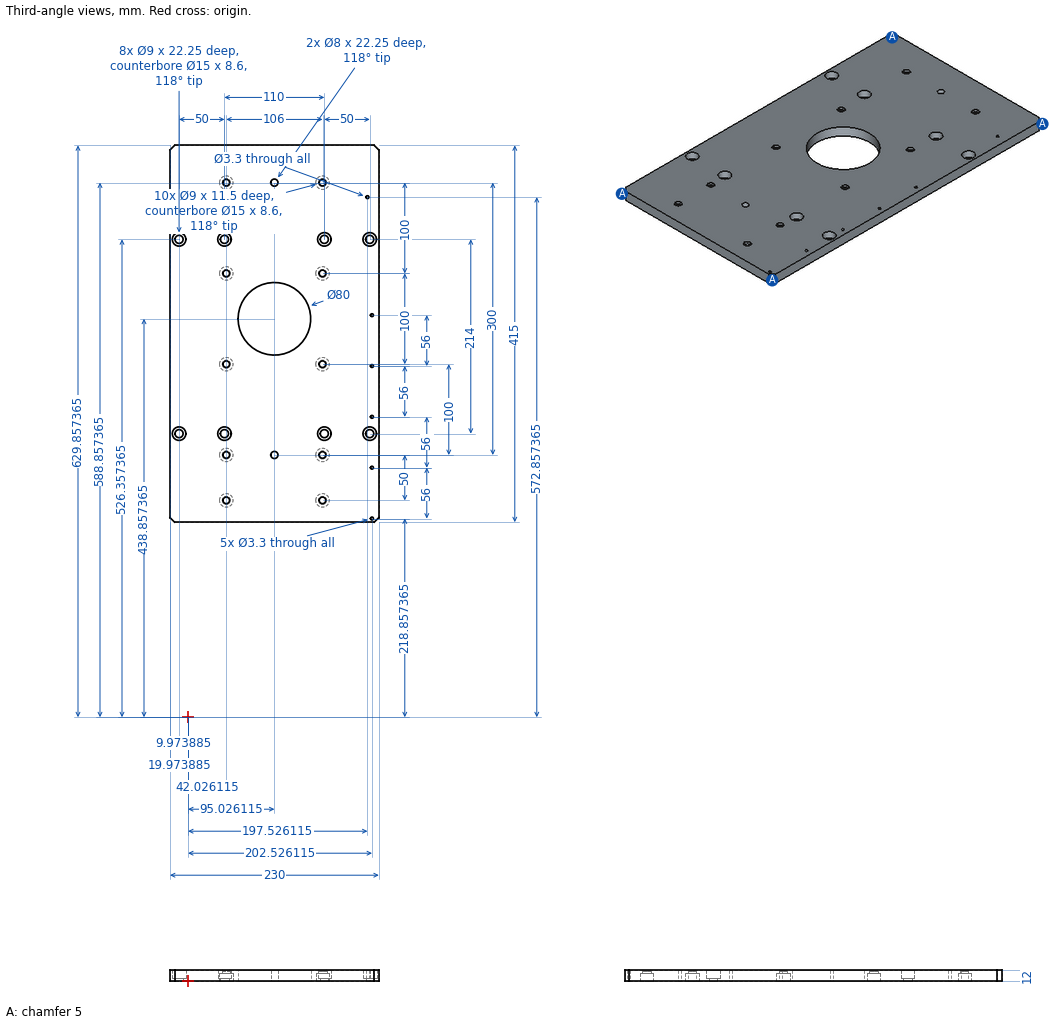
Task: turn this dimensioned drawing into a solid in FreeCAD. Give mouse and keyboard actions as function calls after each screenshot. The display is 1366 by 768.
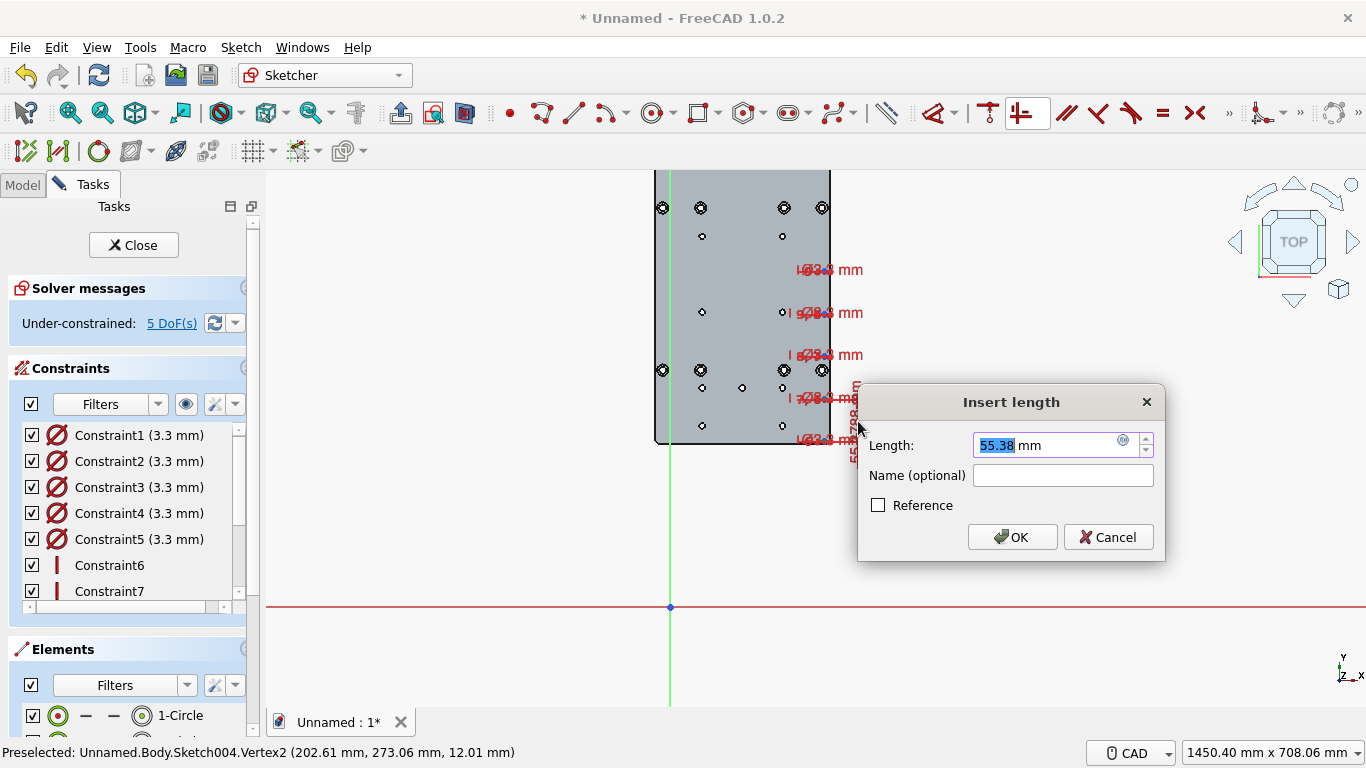
text(56)
key(Return)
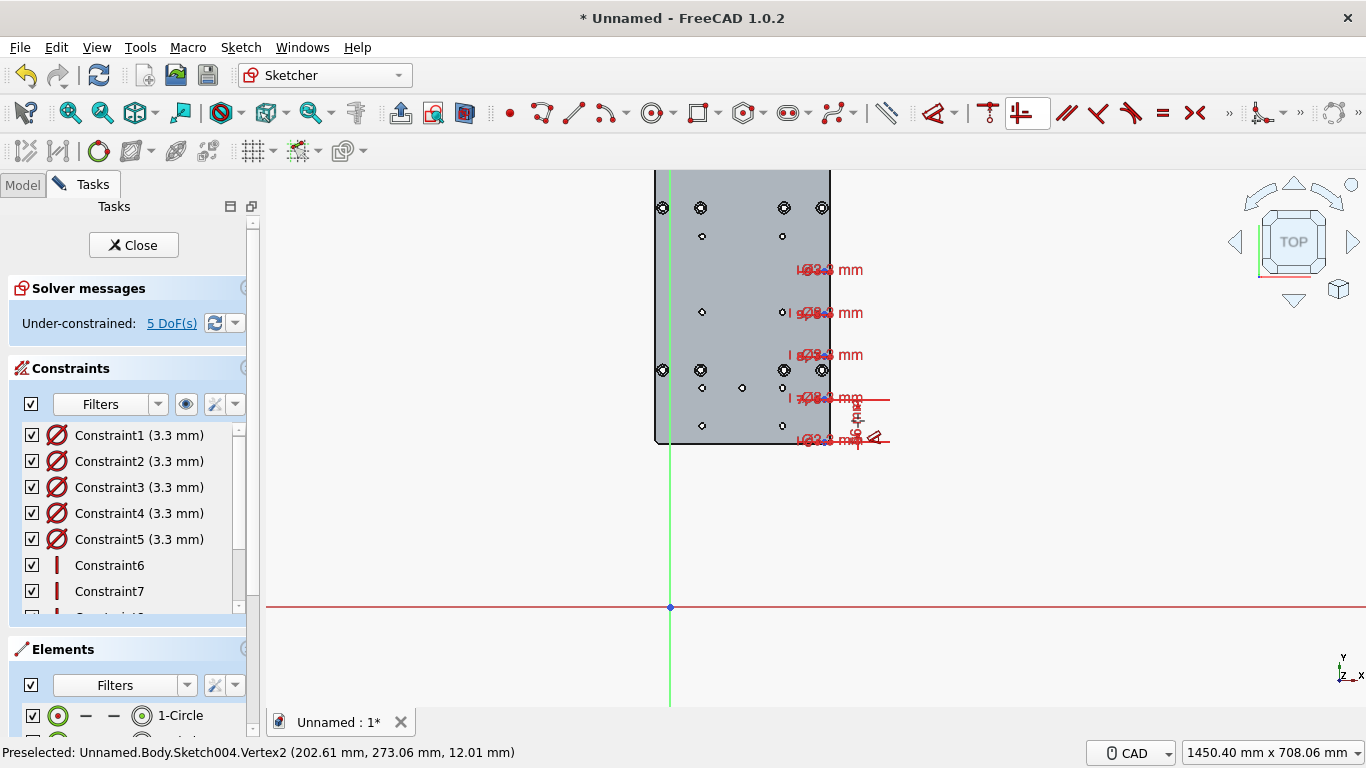
click(824, 400)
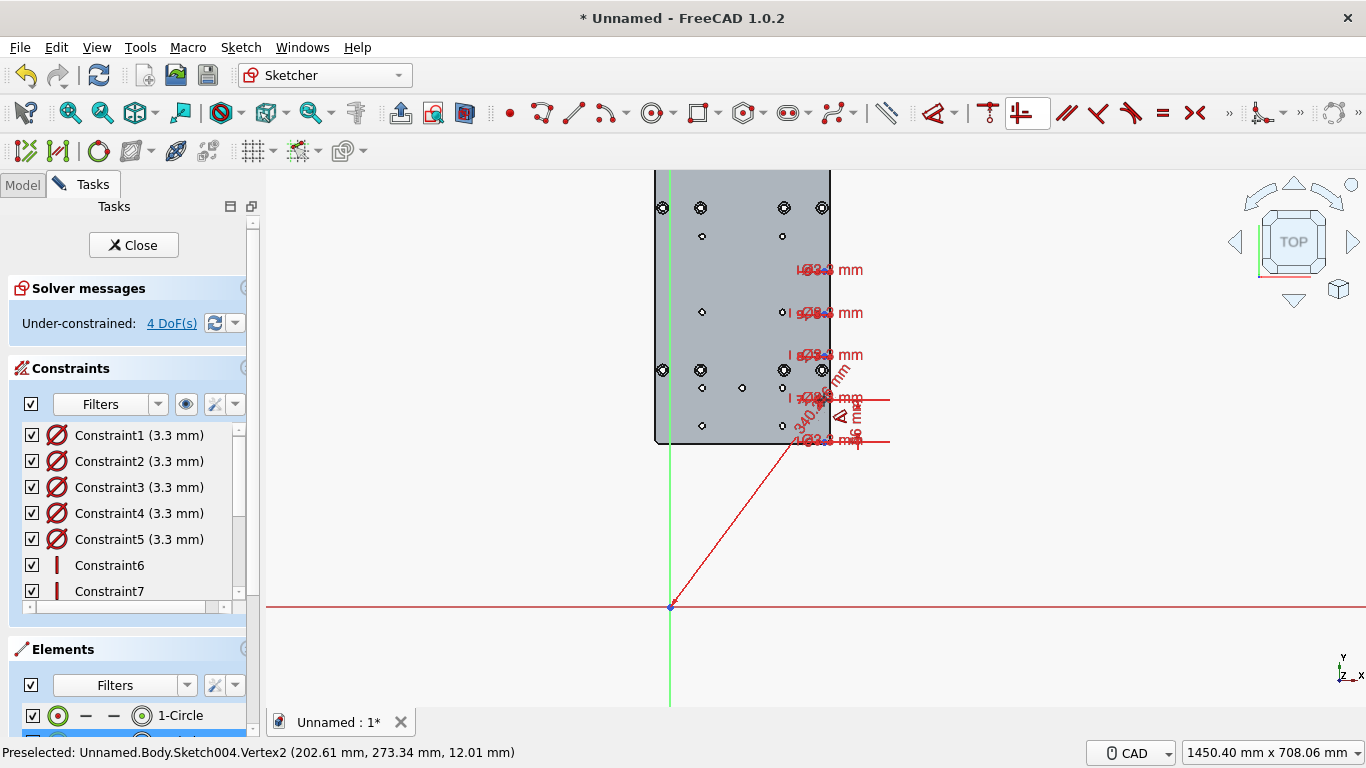
click(824, 357)
click(858, 378)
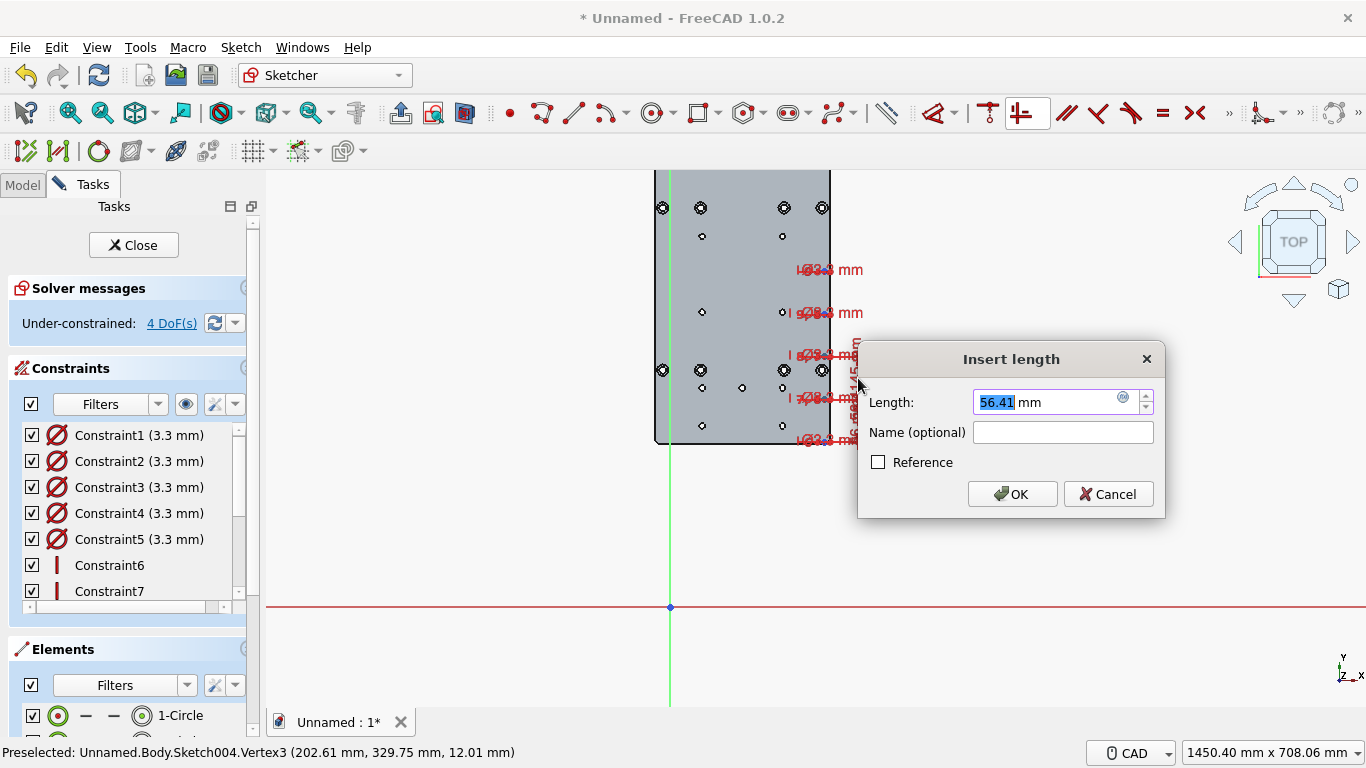
text(56)
key(Return)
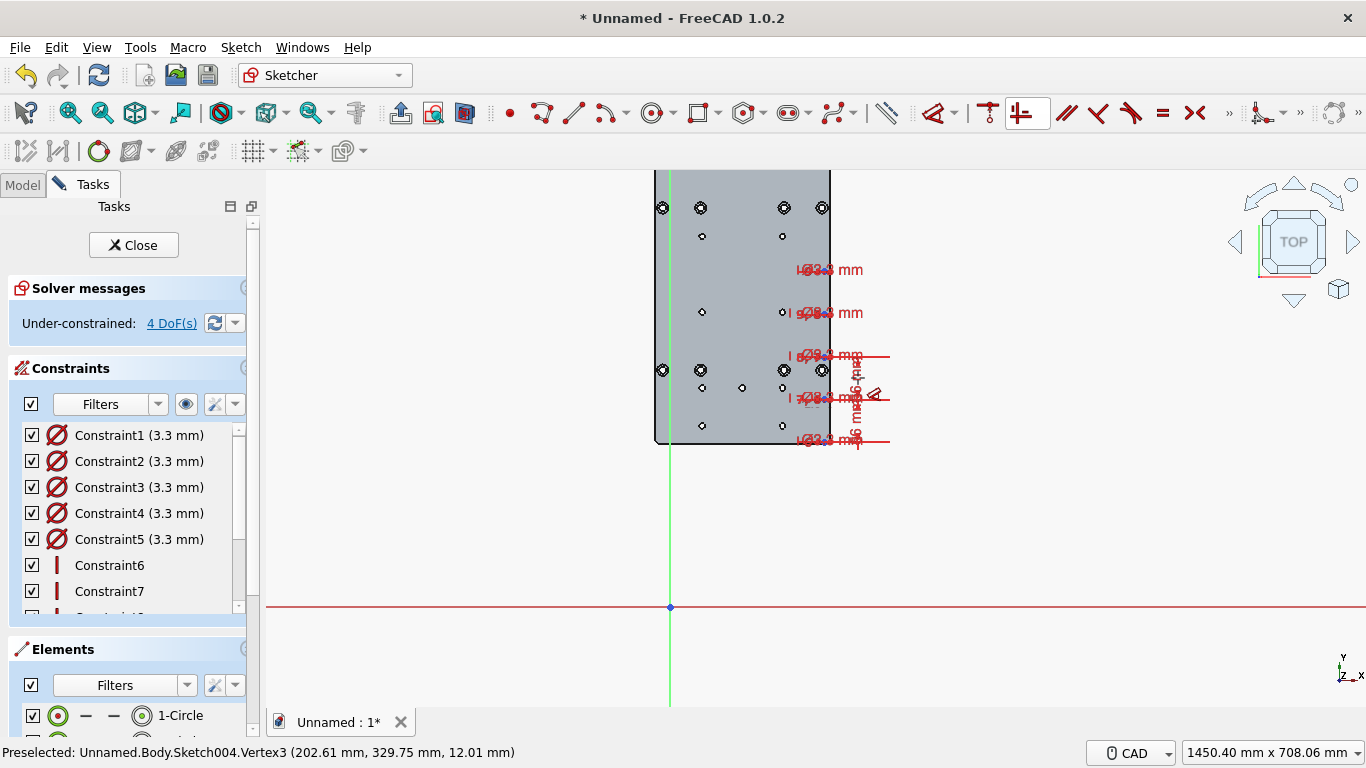
click(824, 357)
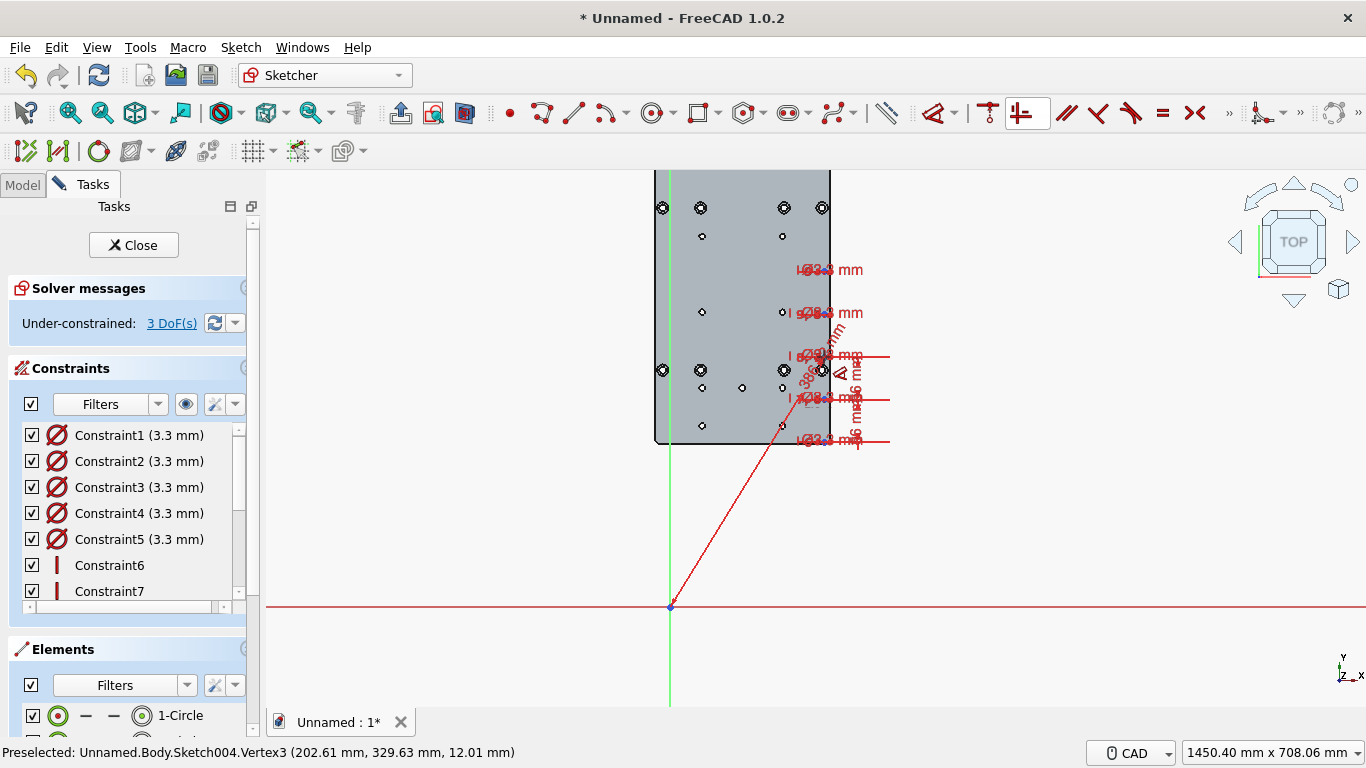
click(824, 315)
click(858, 336)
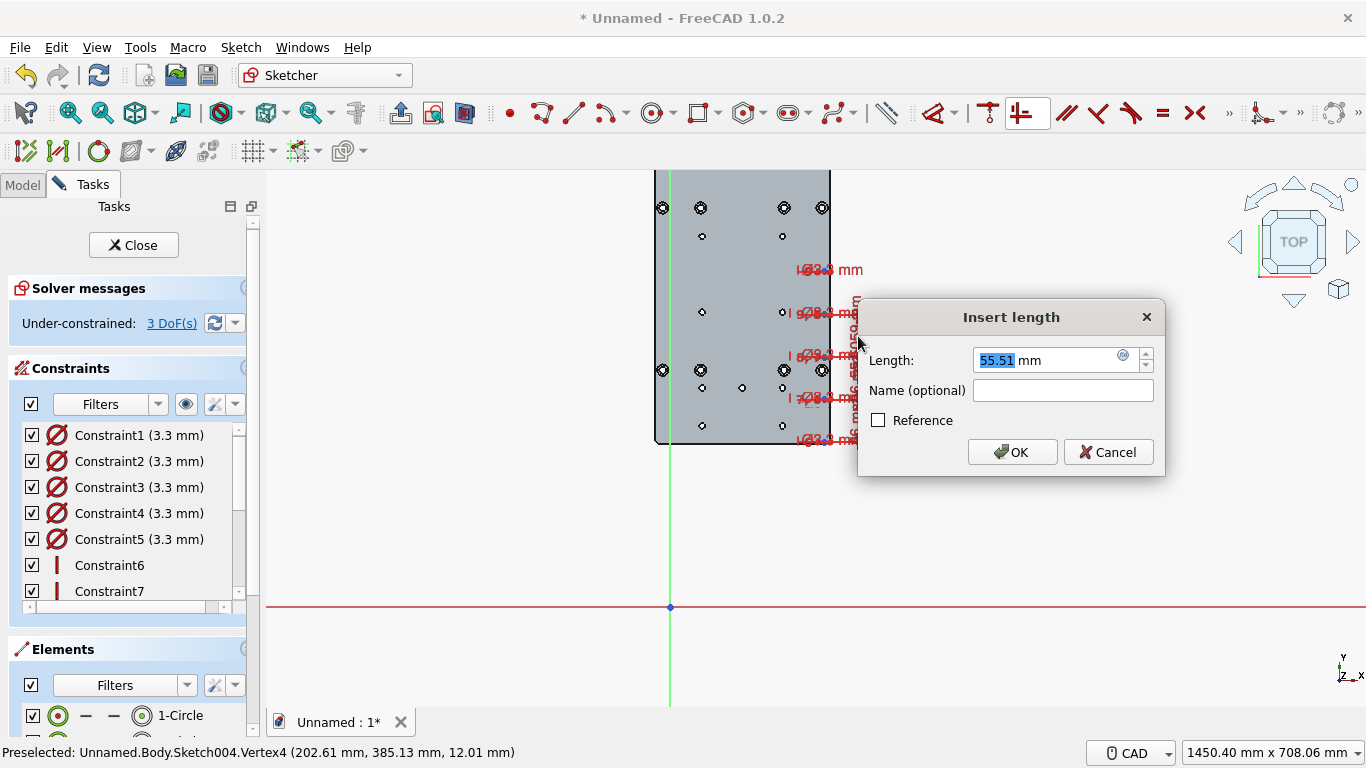
text(56)
key(Return)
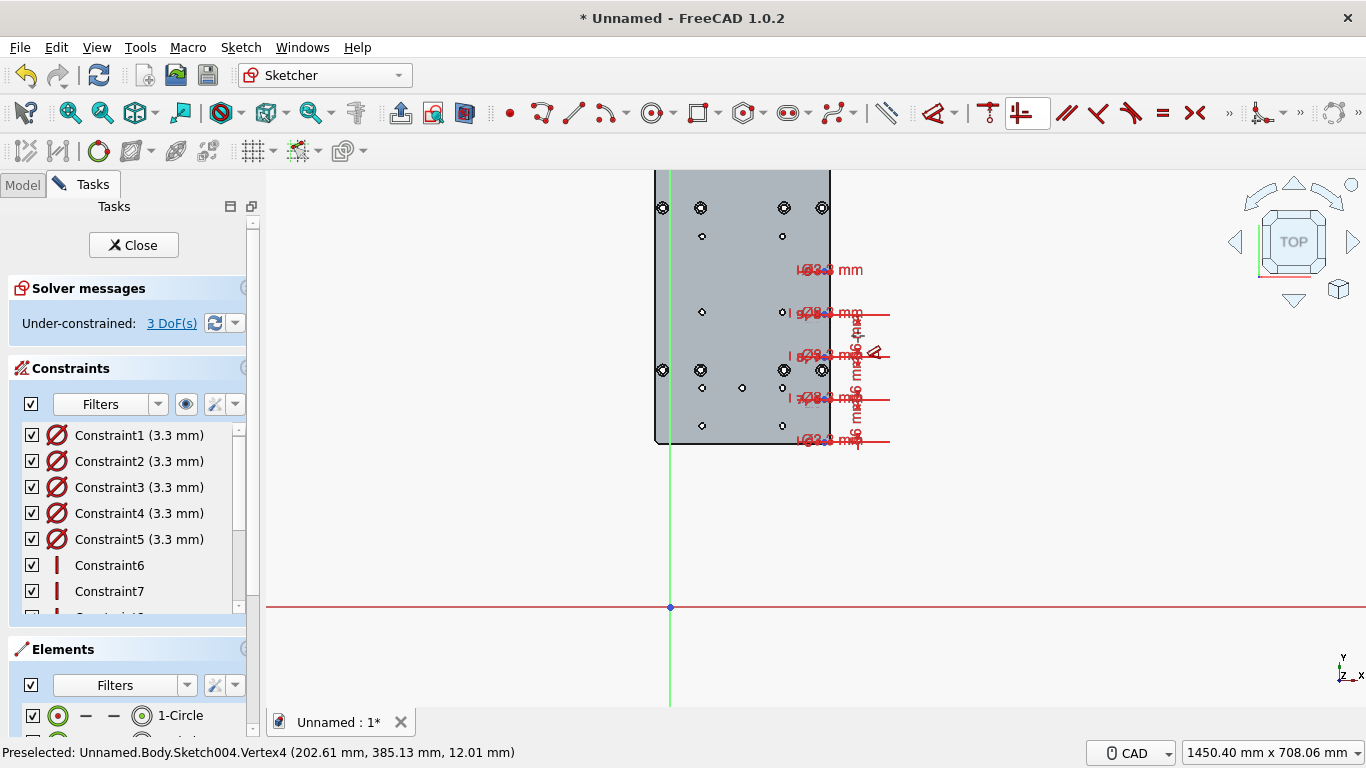
click(824, 315)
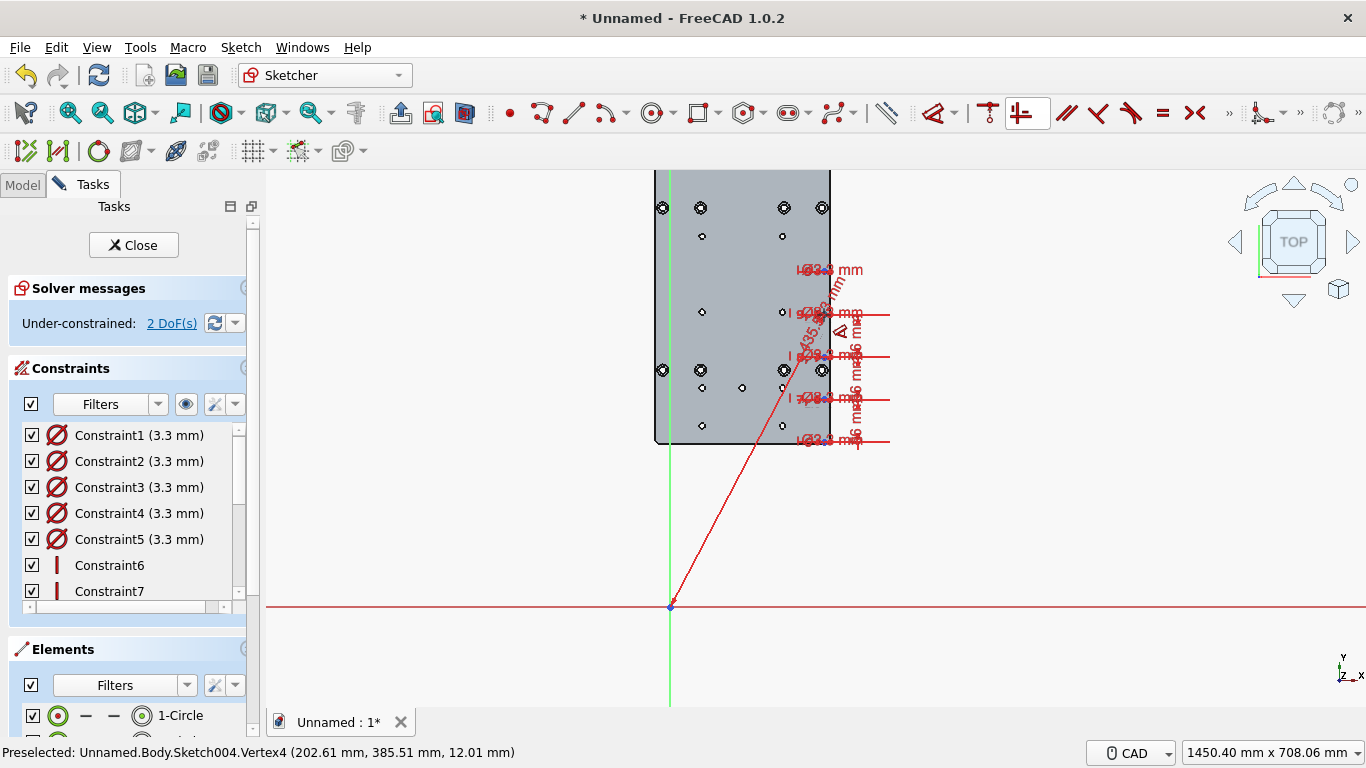
click(824, 272)
click(858, 293)